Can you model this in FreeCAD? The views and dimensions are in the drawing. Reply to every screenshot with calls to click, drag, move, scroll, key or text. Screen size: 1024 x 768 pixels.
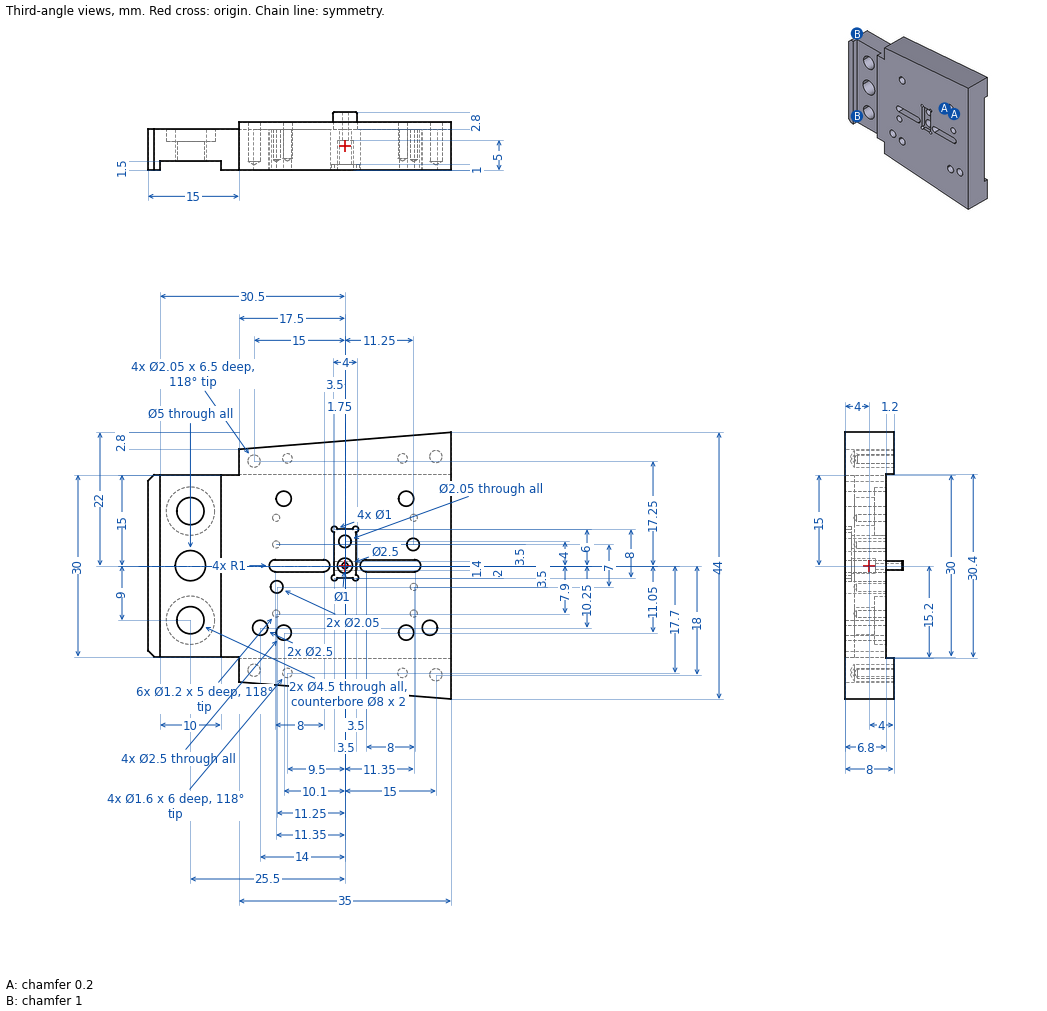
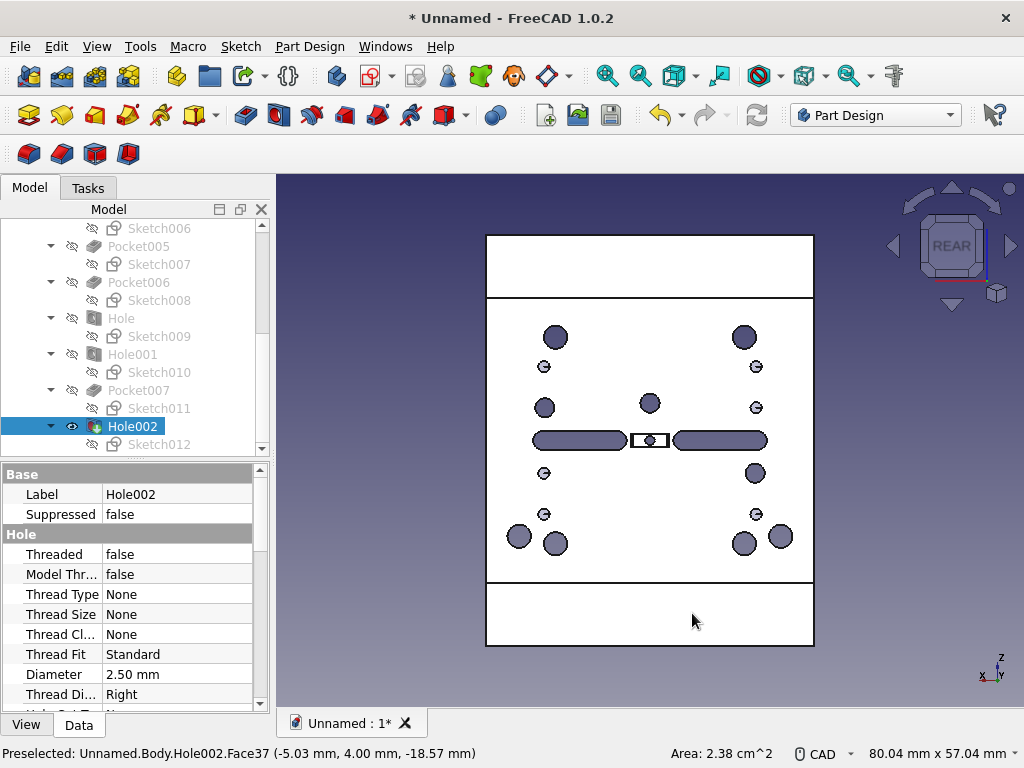
click(370, 76)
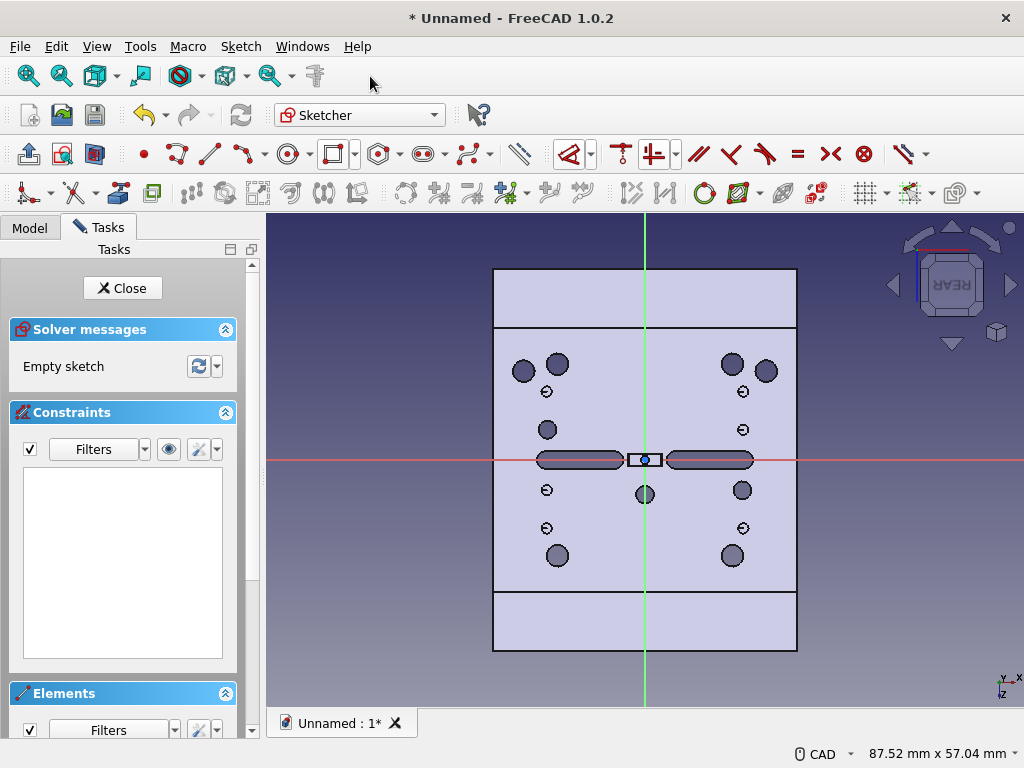
click(177, 154)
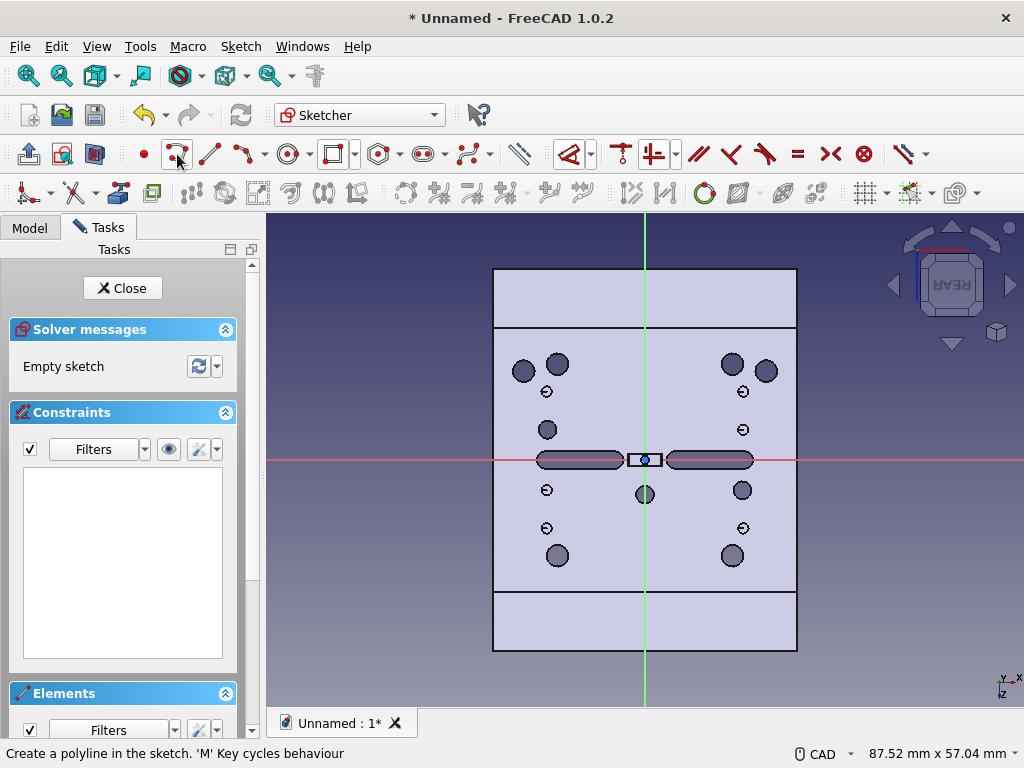
click(493, 626)
click(493, 651)
click(797, 651)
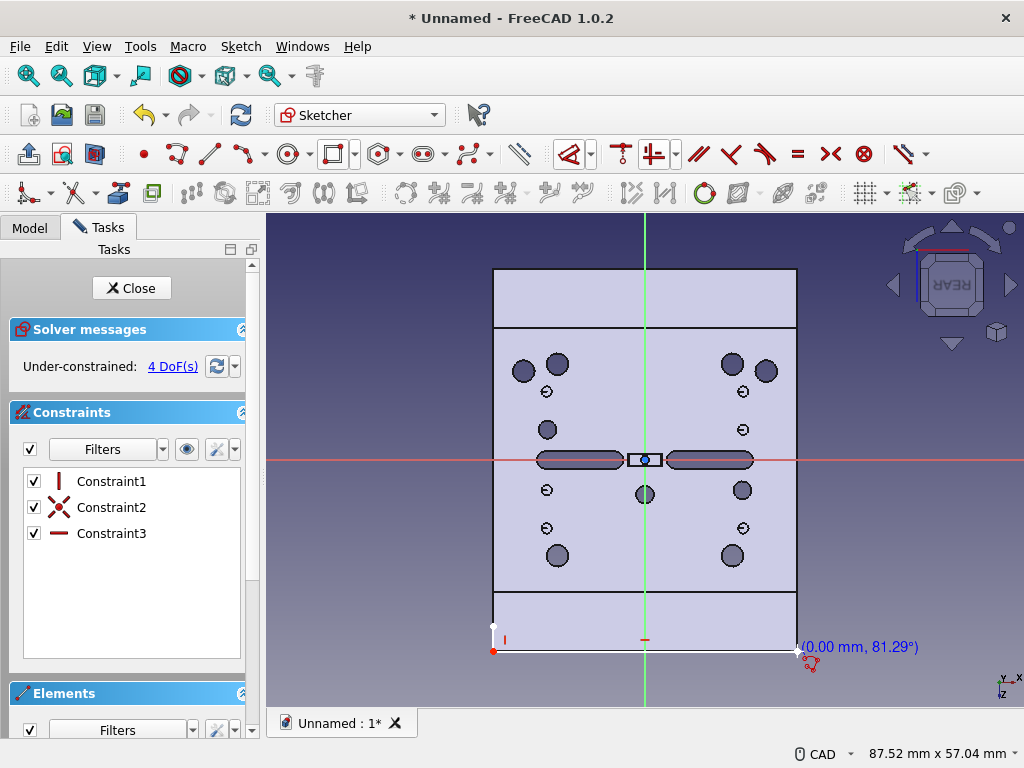
scroll(493, 626, up, 2)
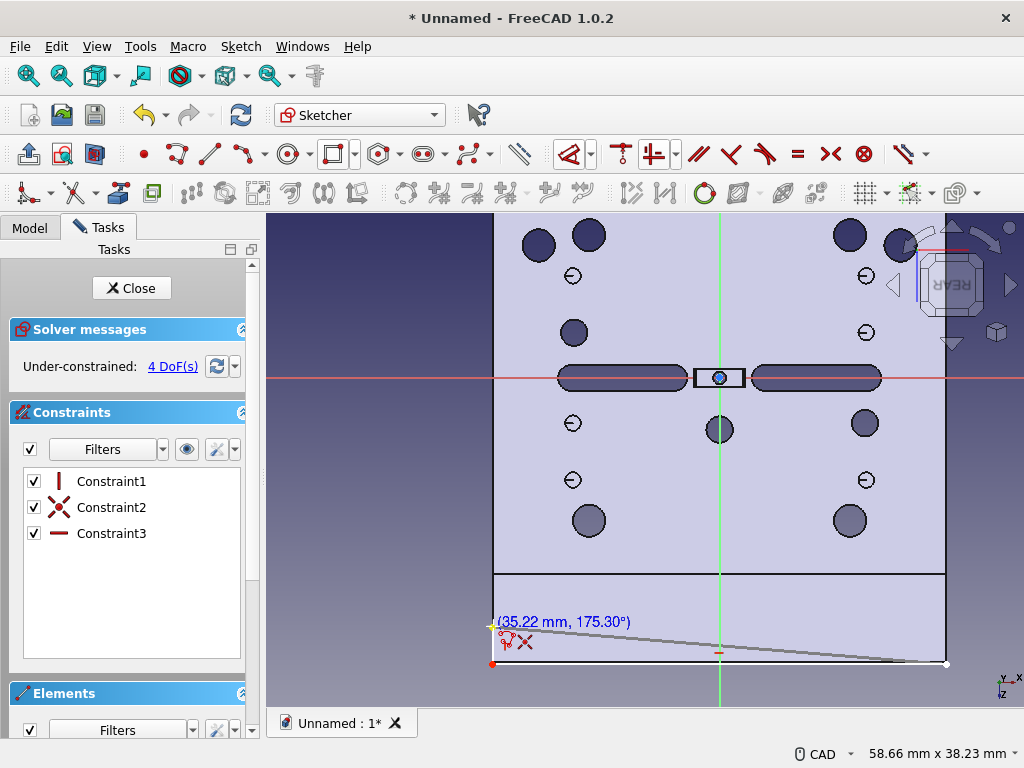
click(493, 627)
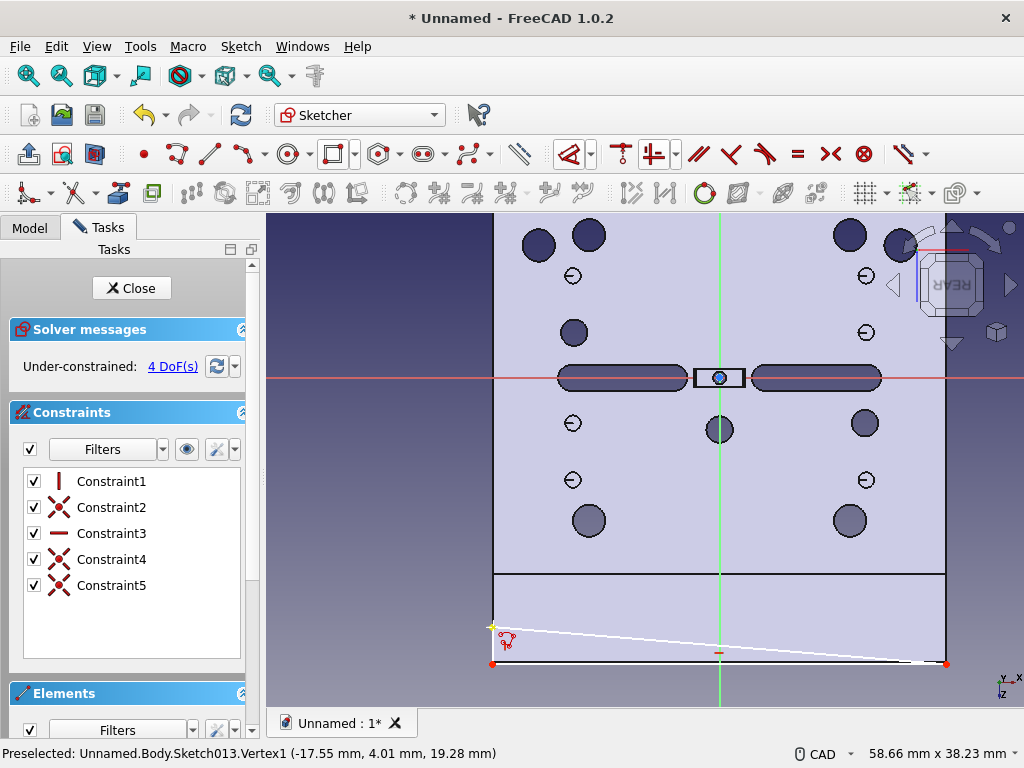
scroll(402, 560, down, 3)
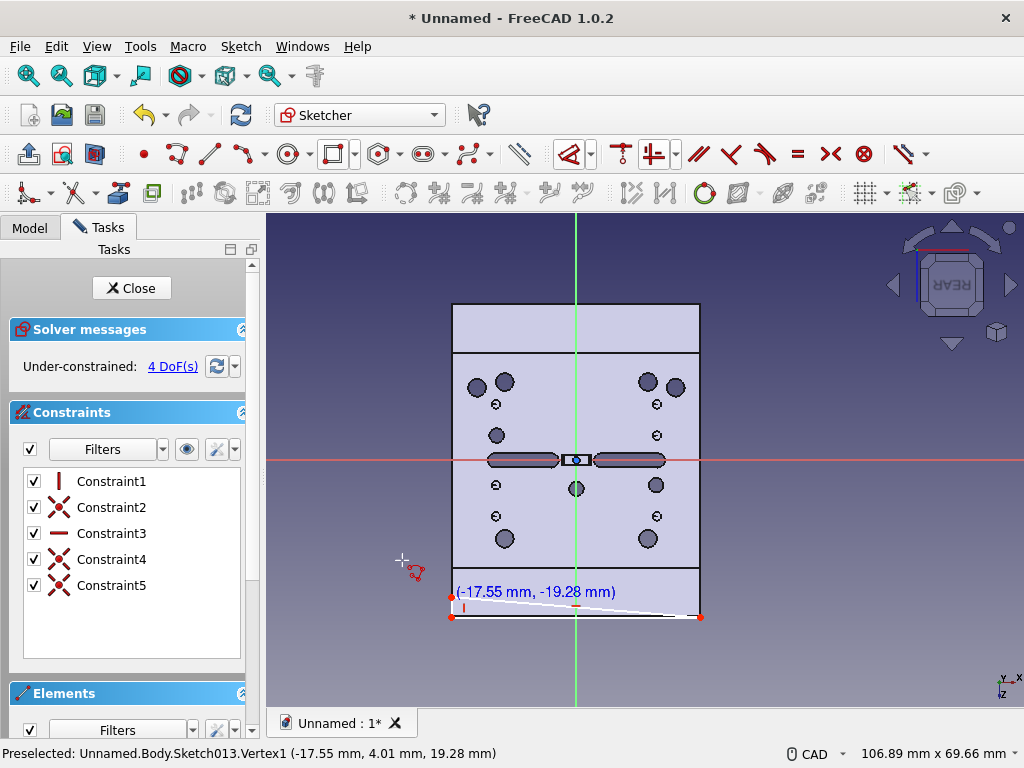
click(452, 324)
click(700, 304)
click(452, 304)
click(452, 325)
key(Escape)
key(Escape)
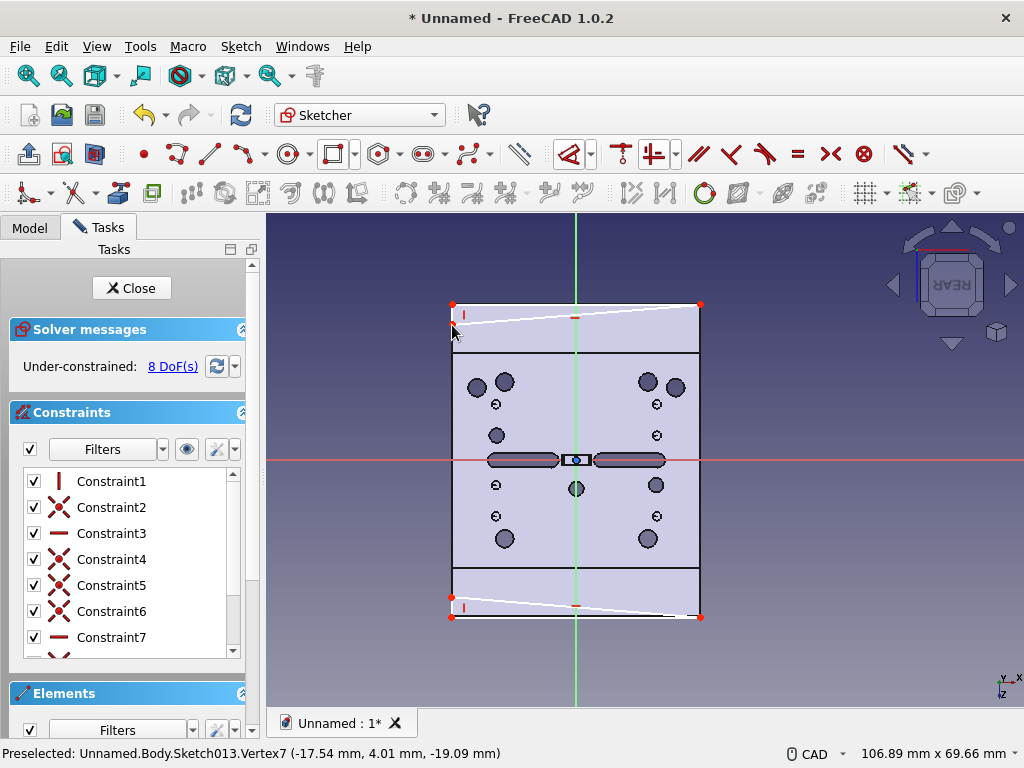
click(452, 597)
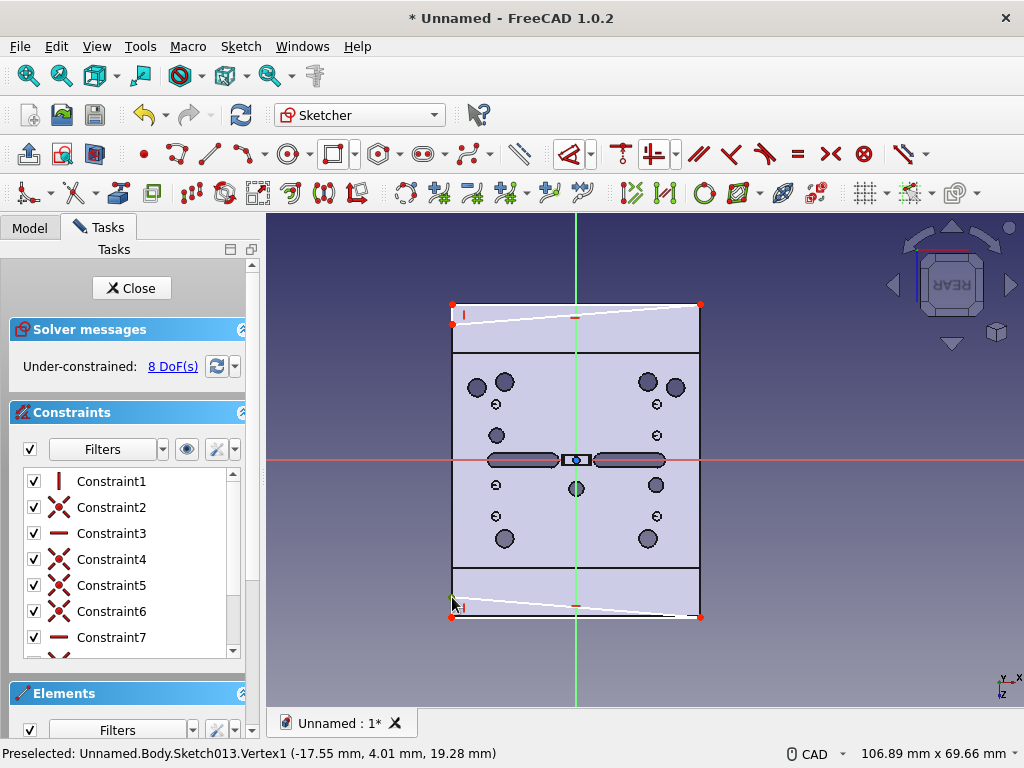
click(452, 325)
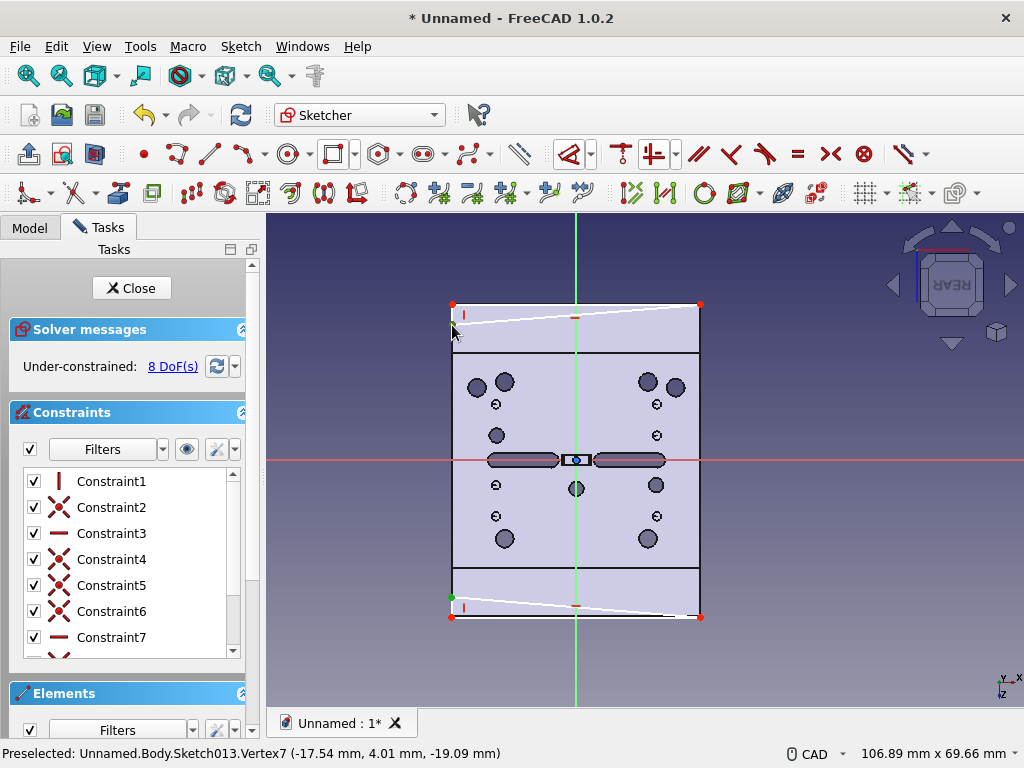
click(334, 460)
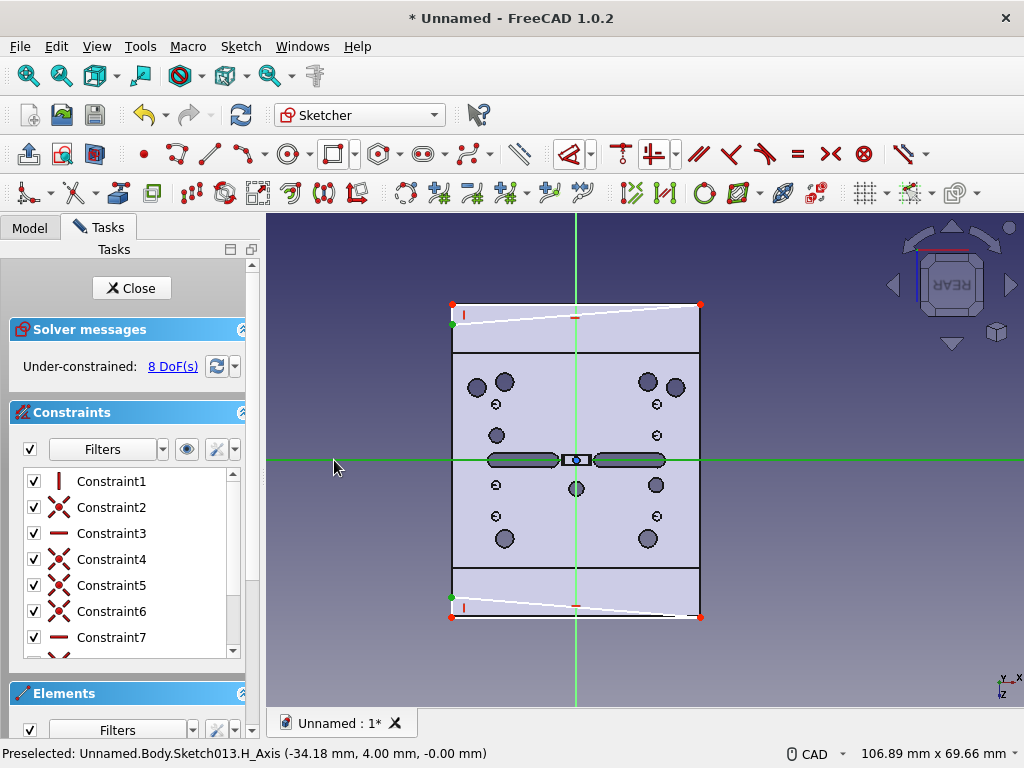
click(831, 154)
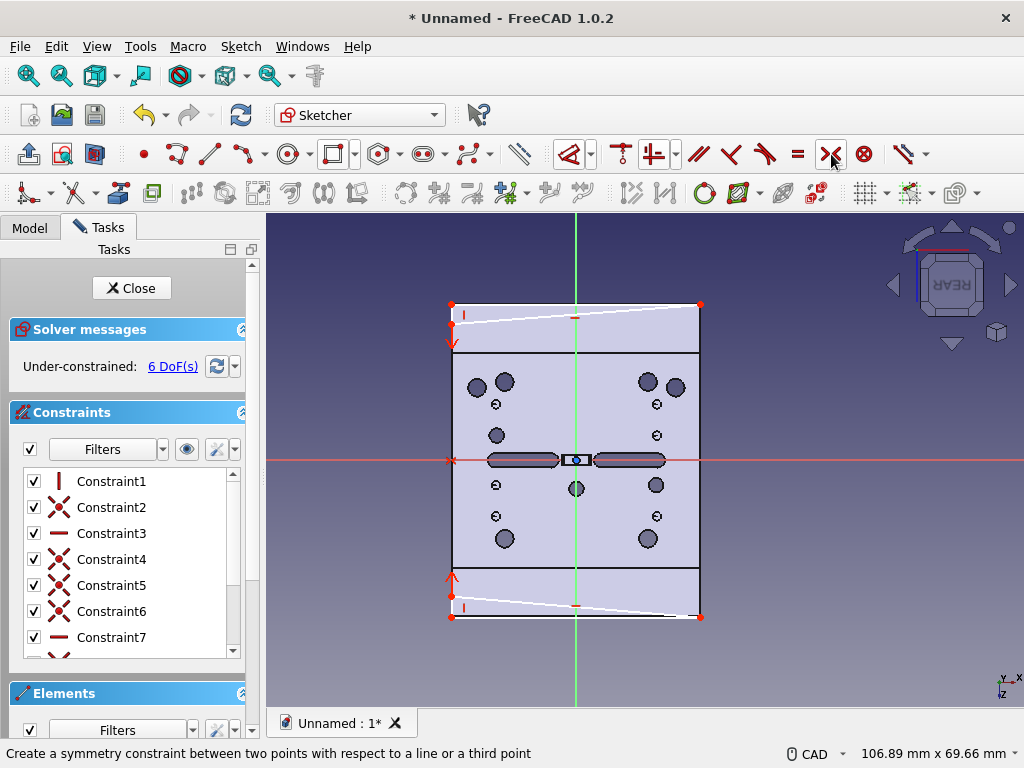
click(701, 618)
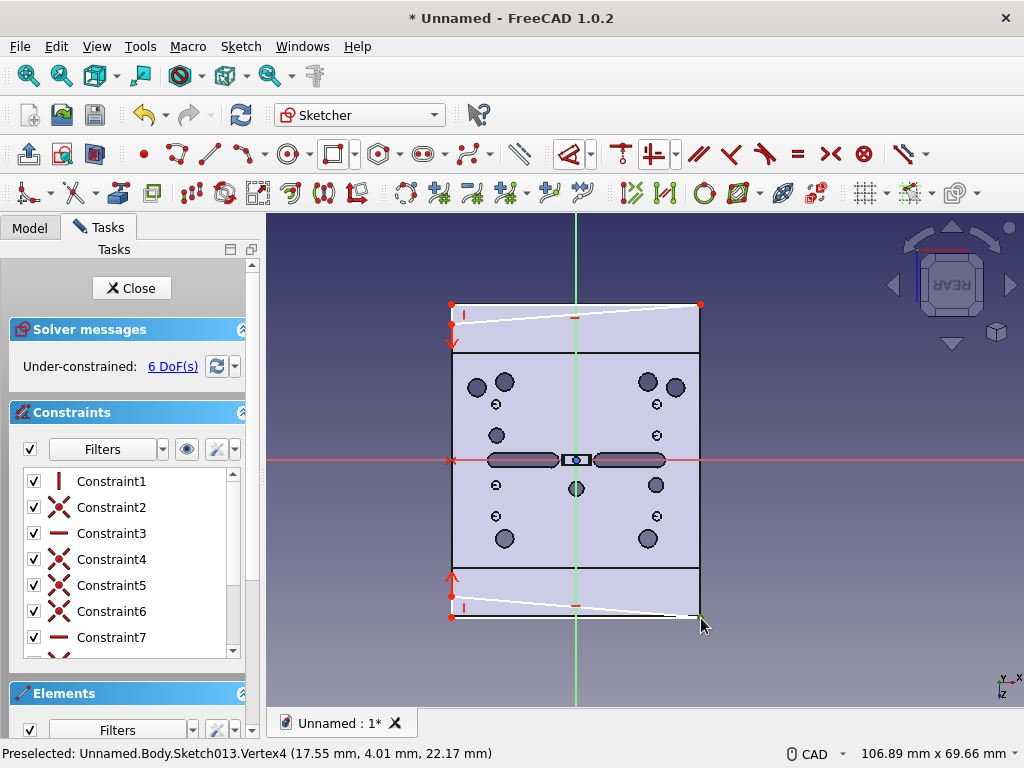
click(700, 305)